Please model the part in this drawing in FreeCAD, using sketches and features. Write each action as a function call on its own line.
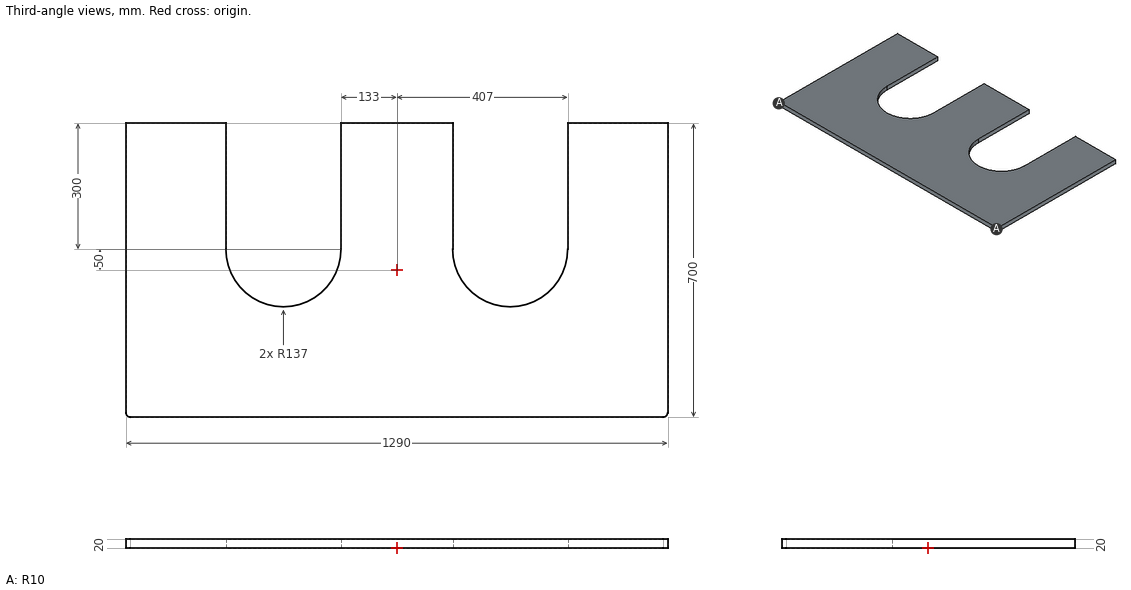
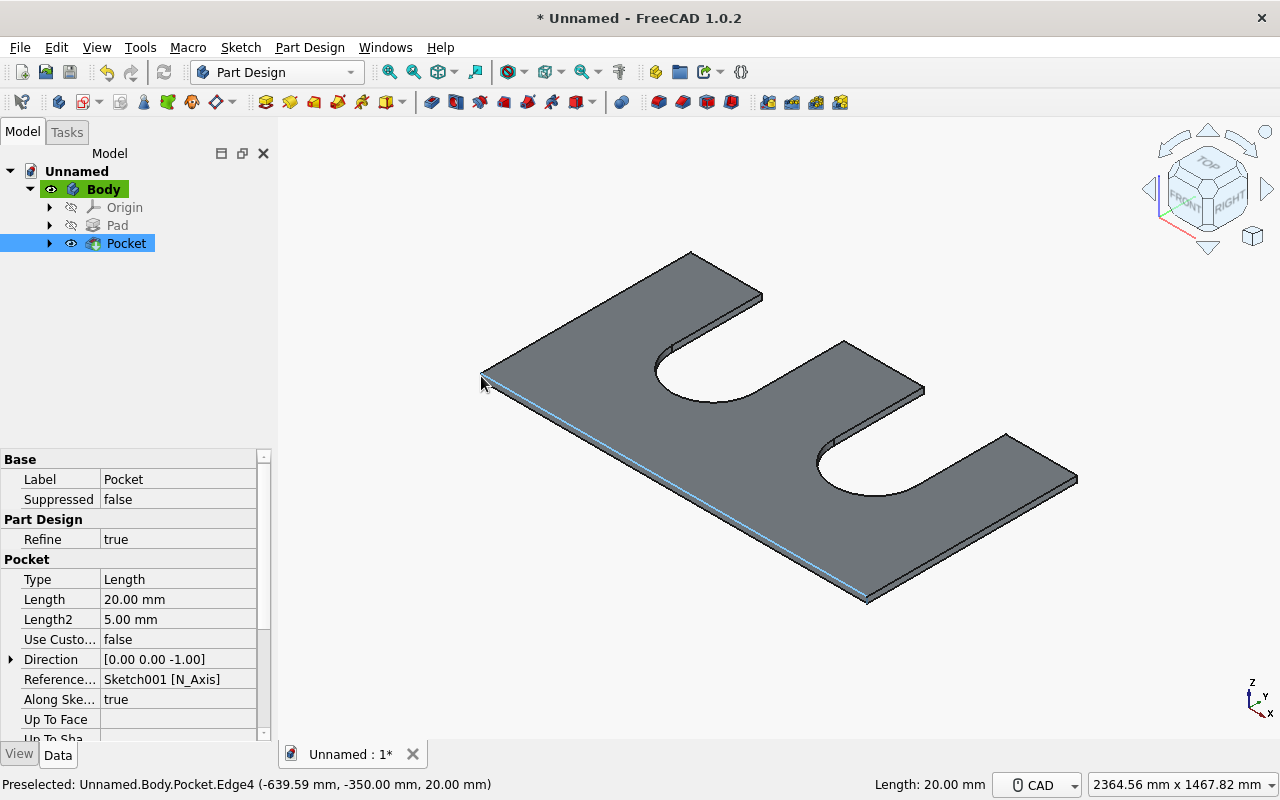
key(2)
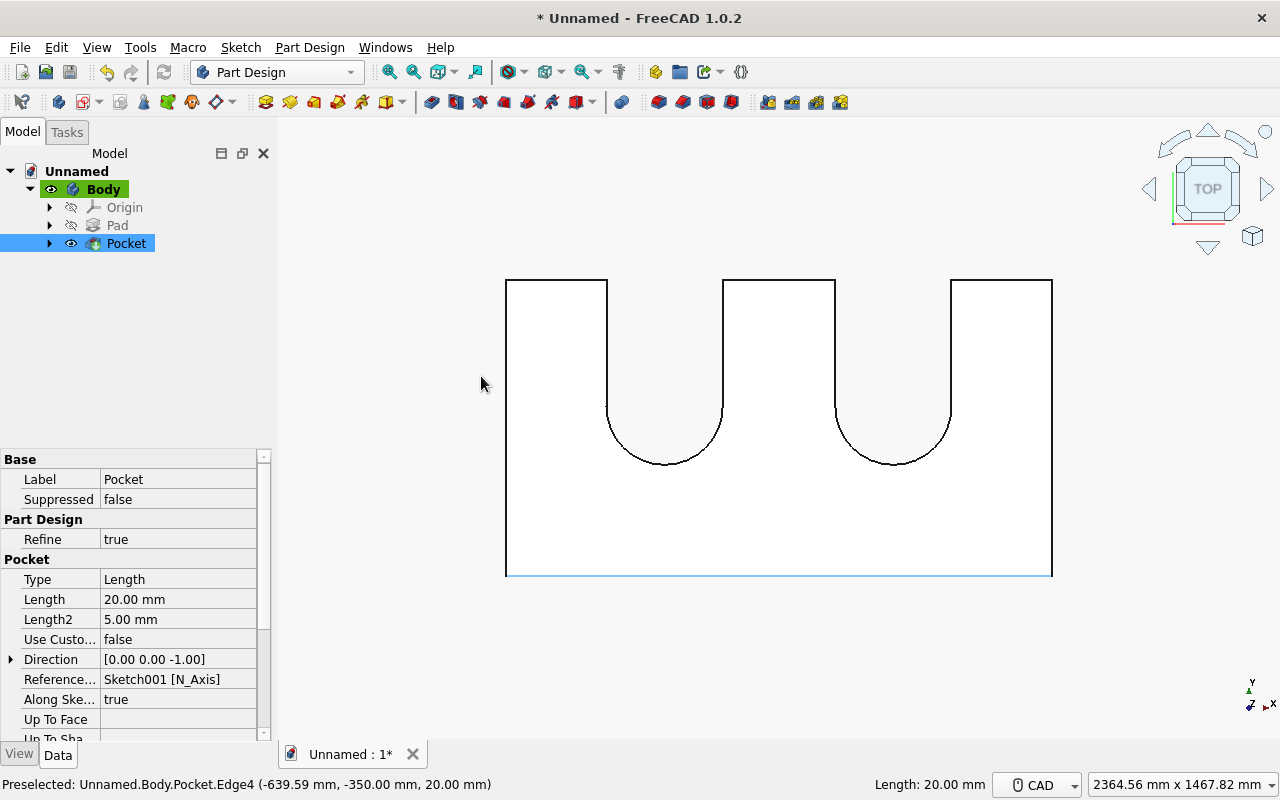
scroll(506, 575, up, 8)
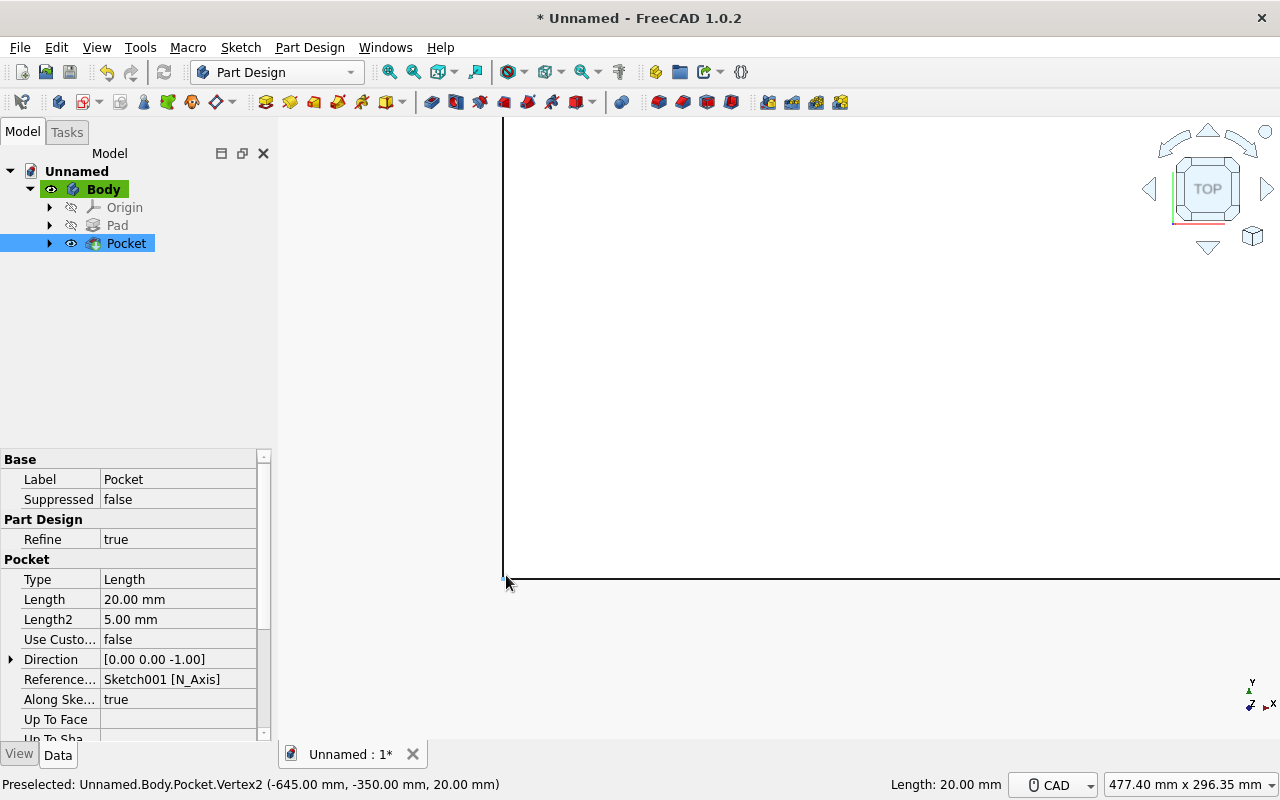
key(v)
key(f)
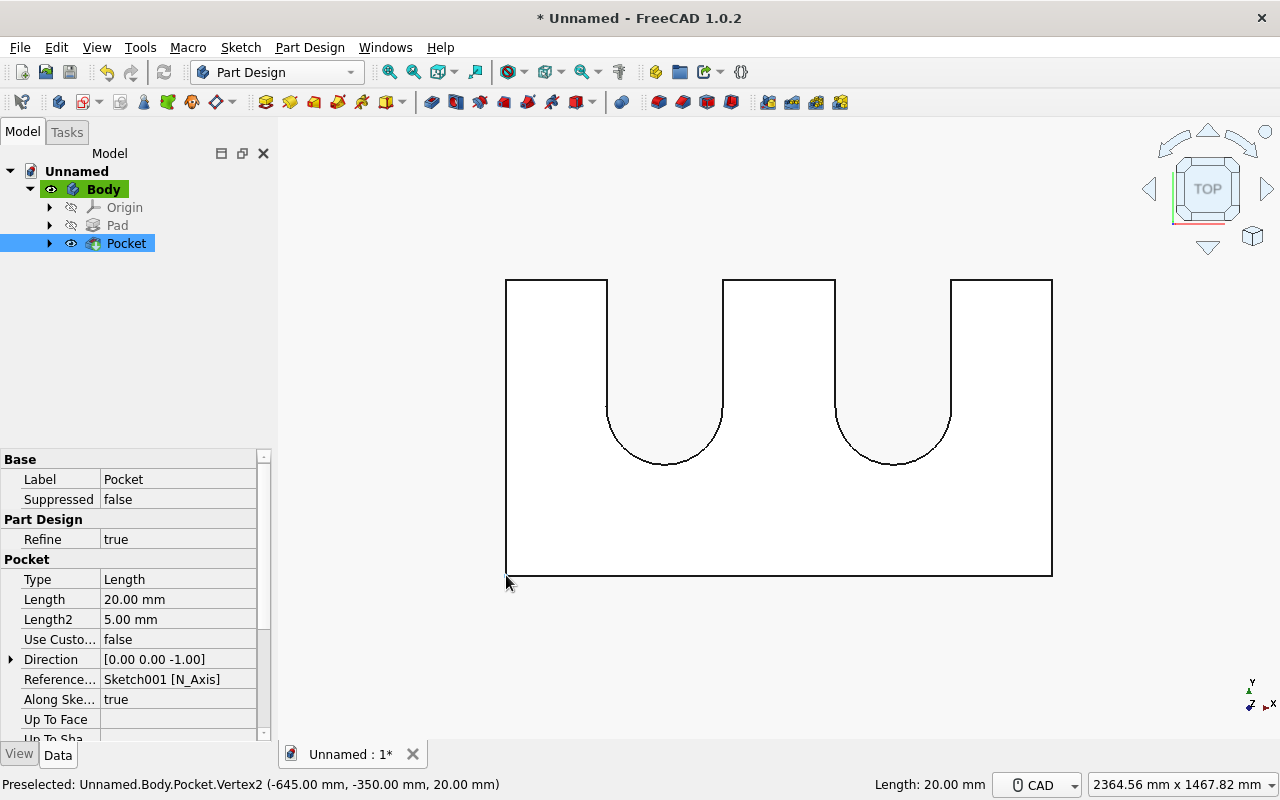
key(1)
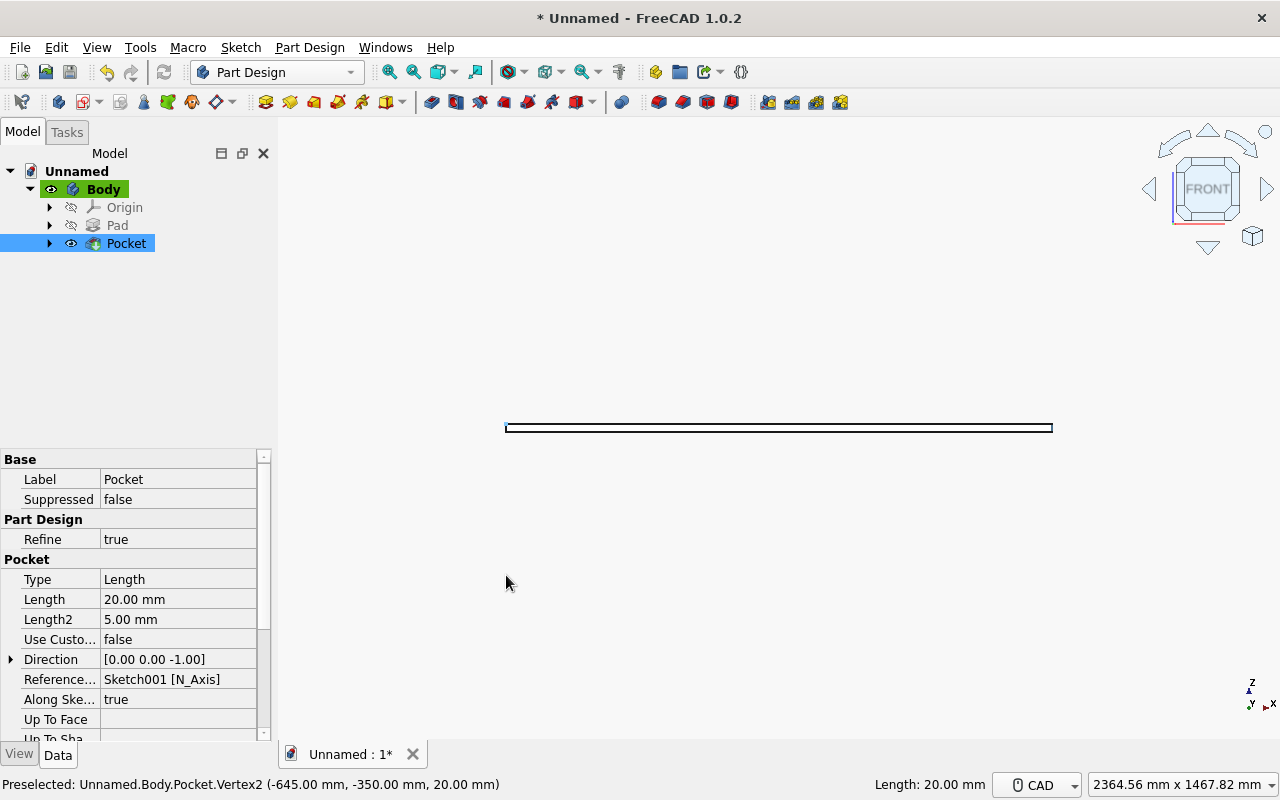
scroll(506, 427, up, 8)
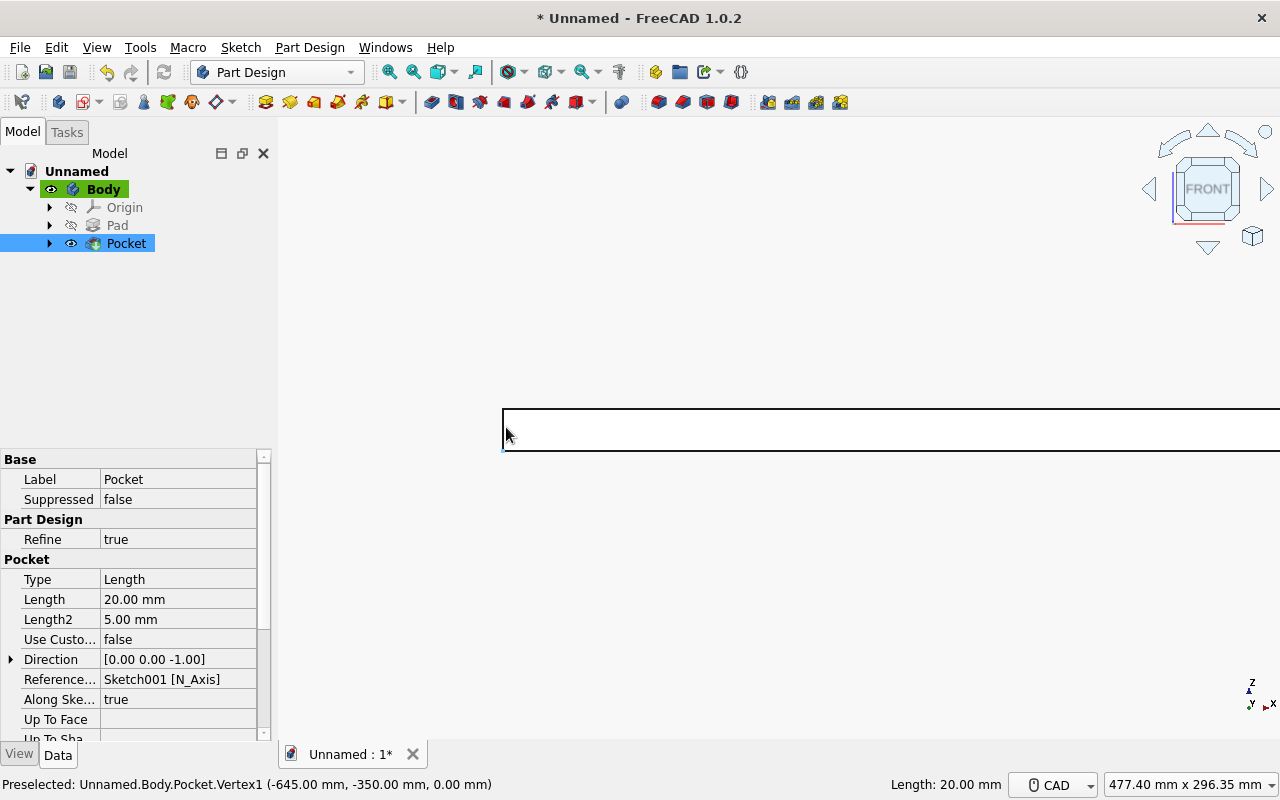
click(503, 429, ctrl)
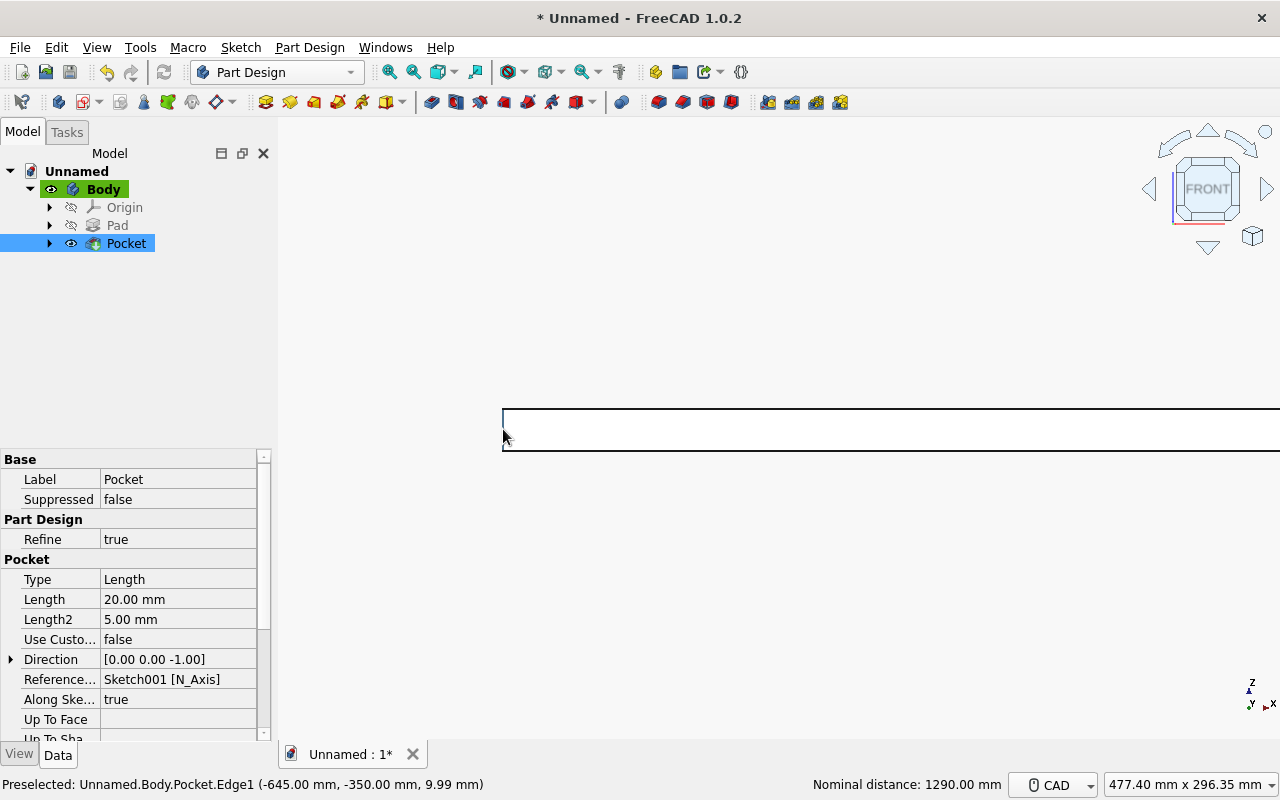
click(660, 102)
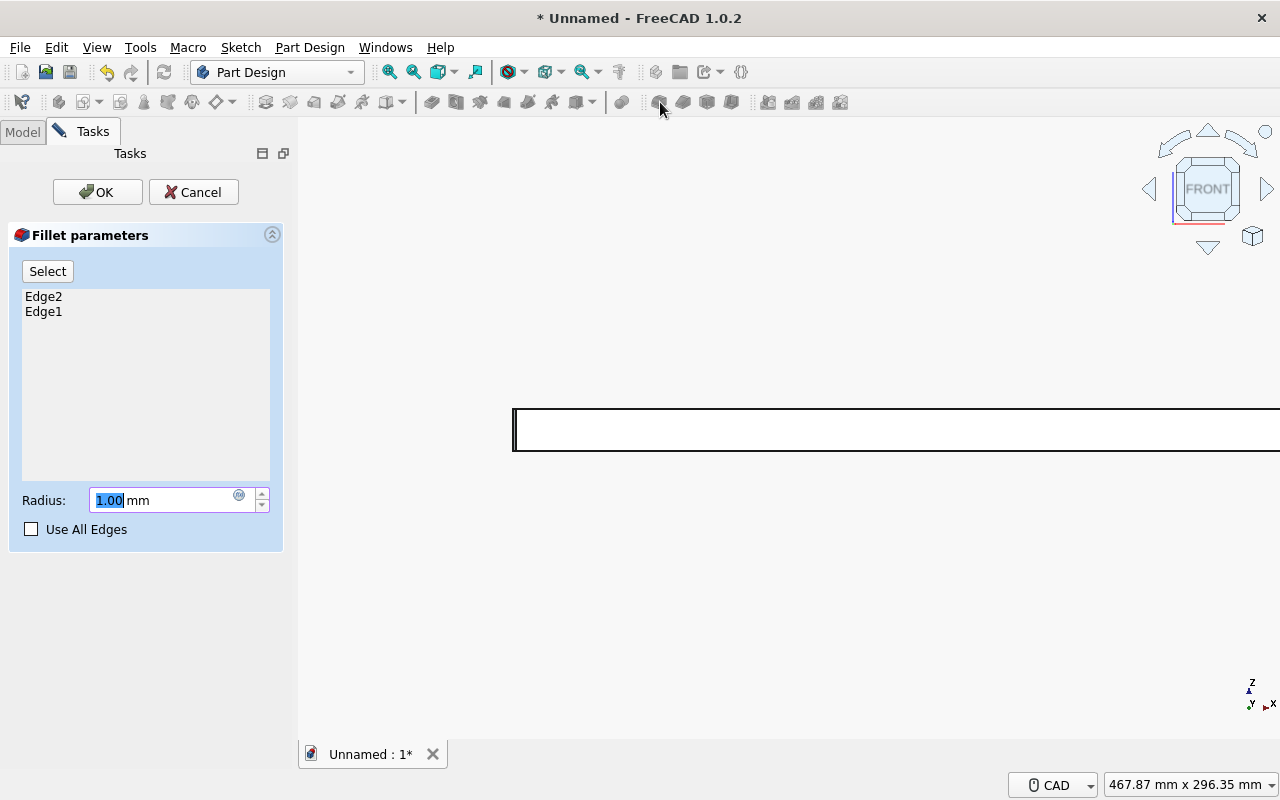
text(10)
key(Tab)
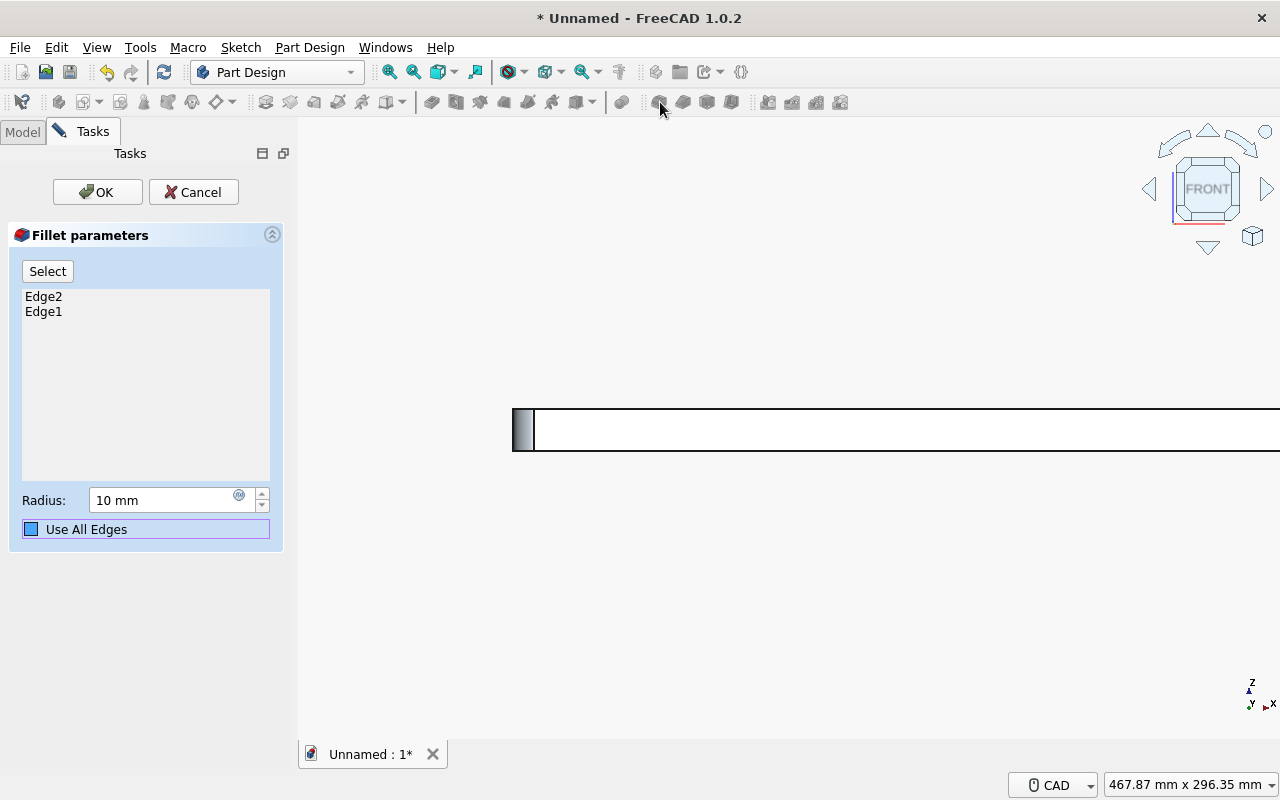
click(98, 192)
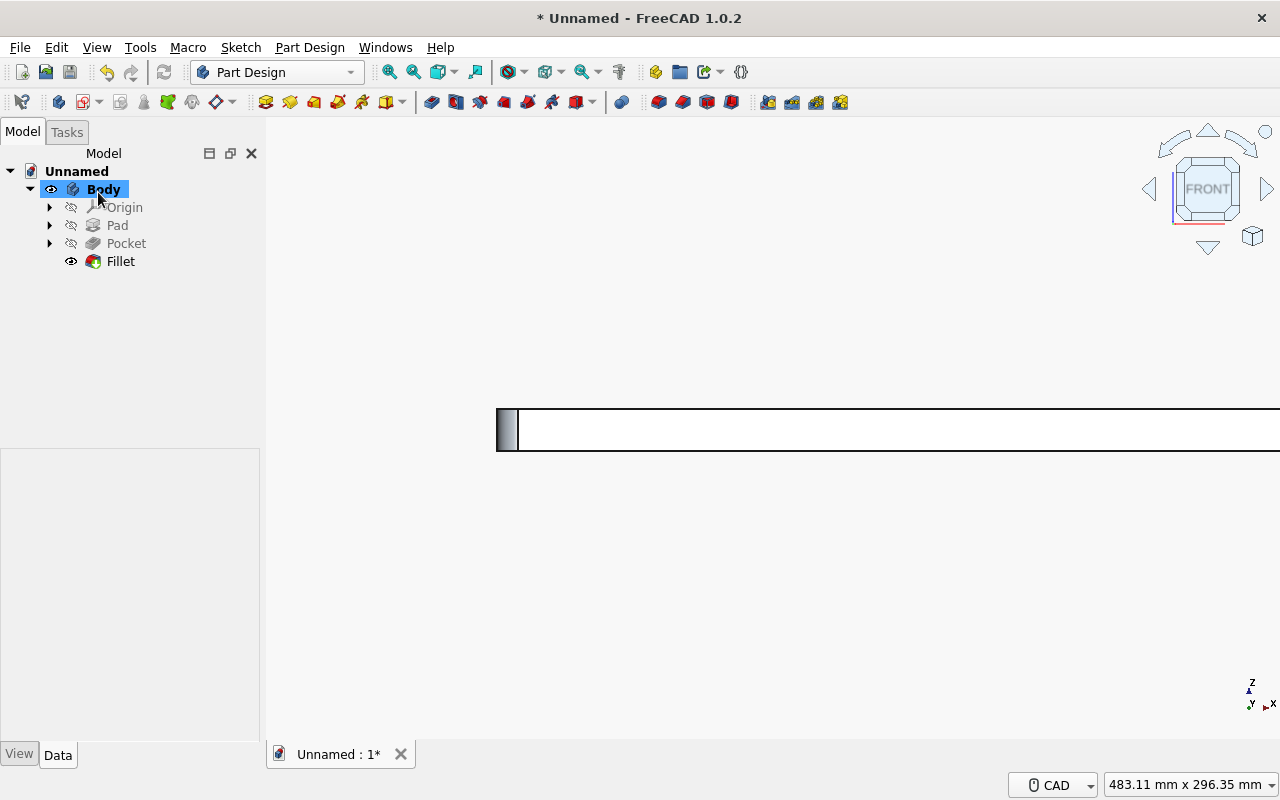
key(0)